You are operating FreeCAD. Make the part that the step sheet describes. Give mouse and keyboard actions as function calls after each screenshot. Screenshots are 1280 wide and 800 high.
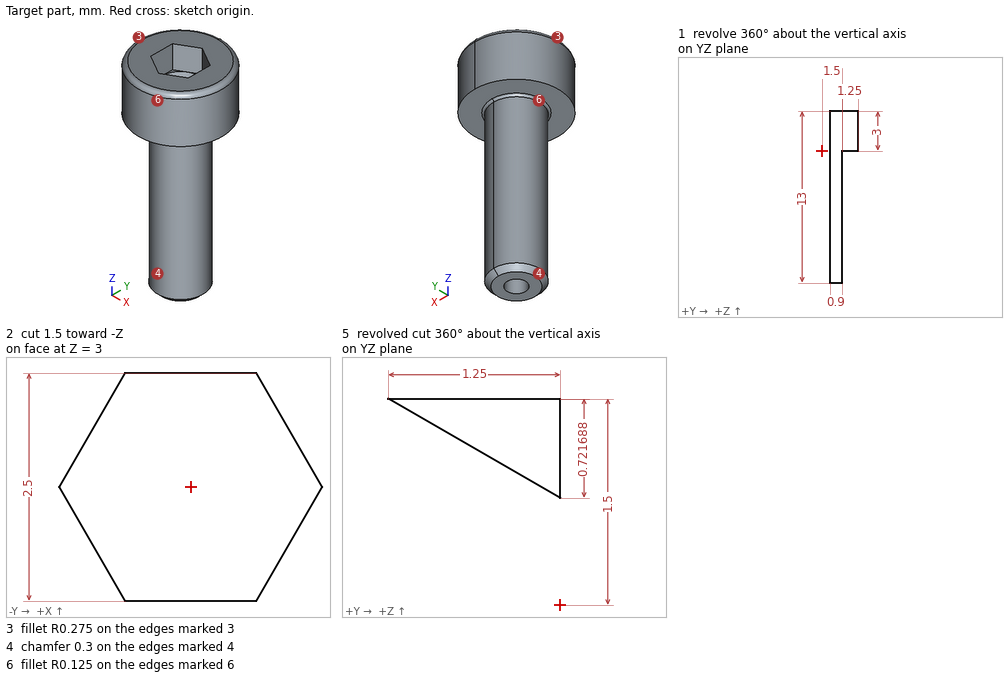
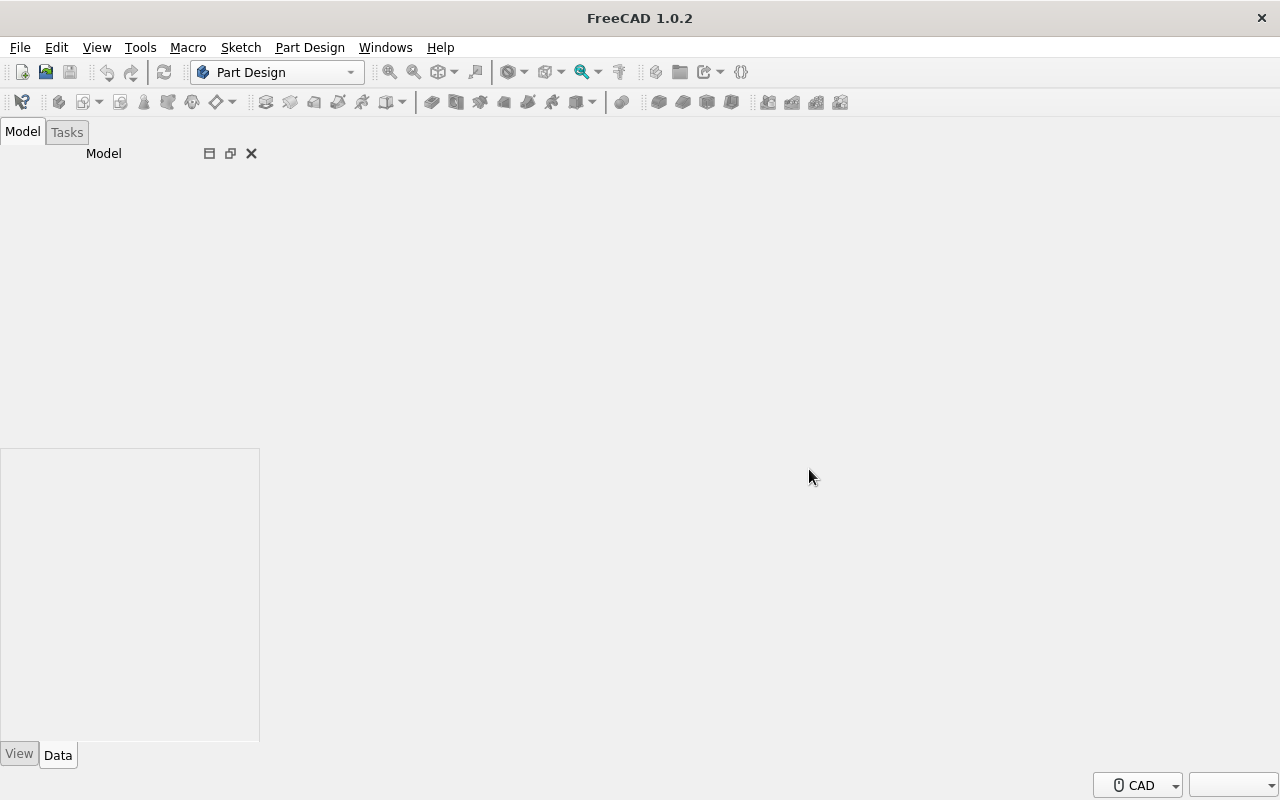
click(22, 72)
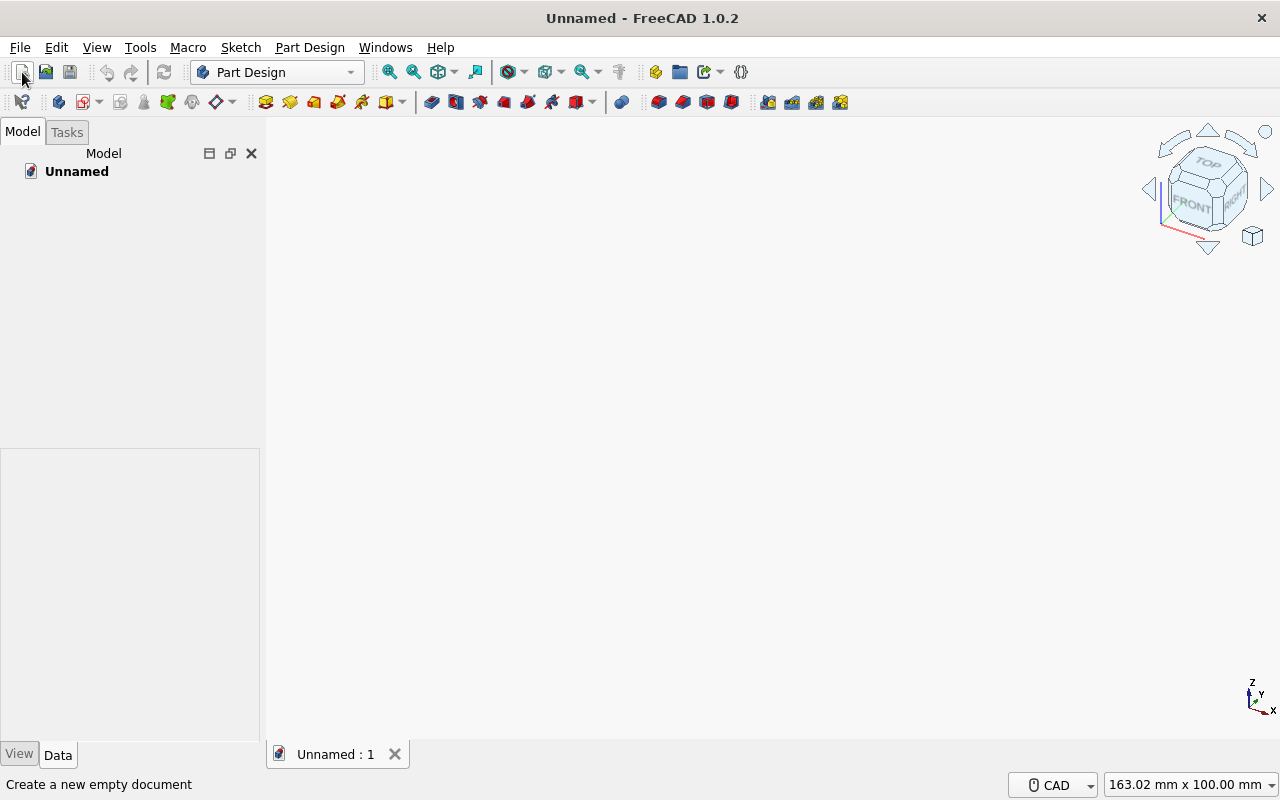
click(84, 102)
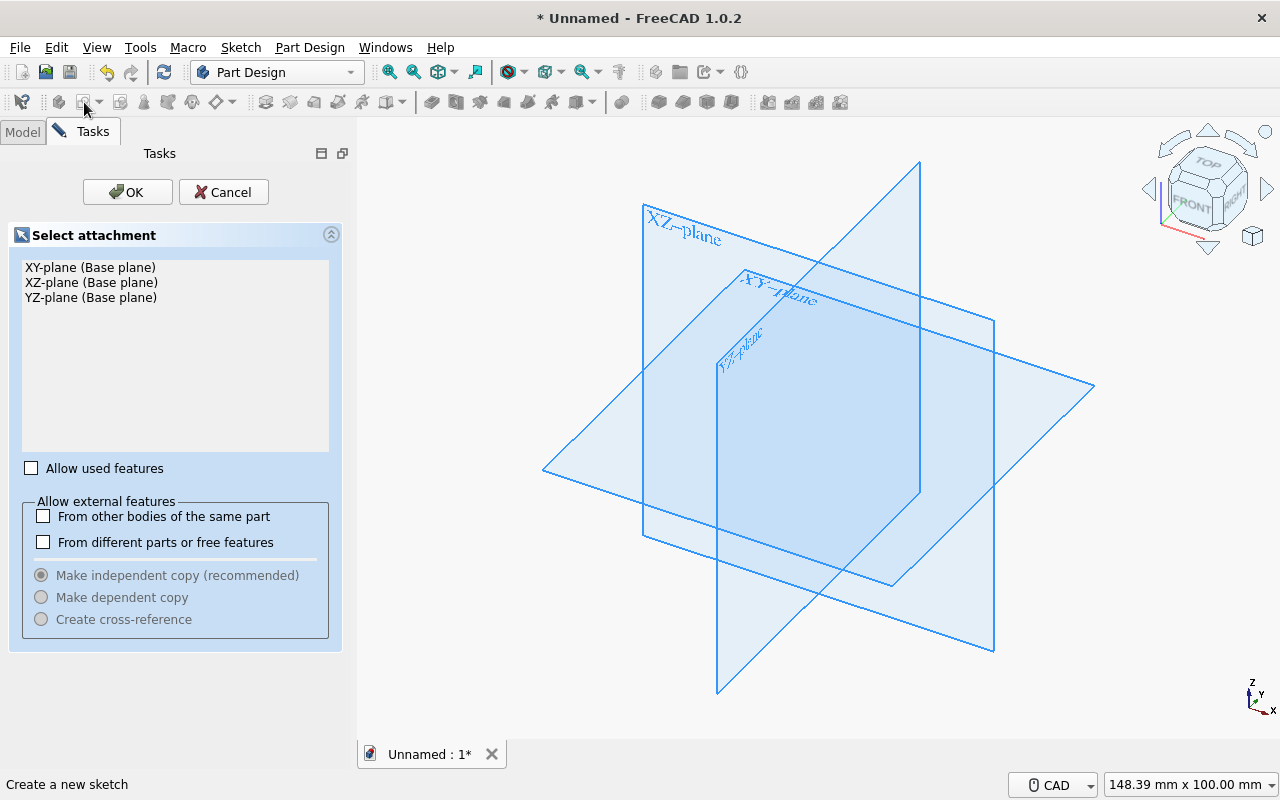
click(82, 298)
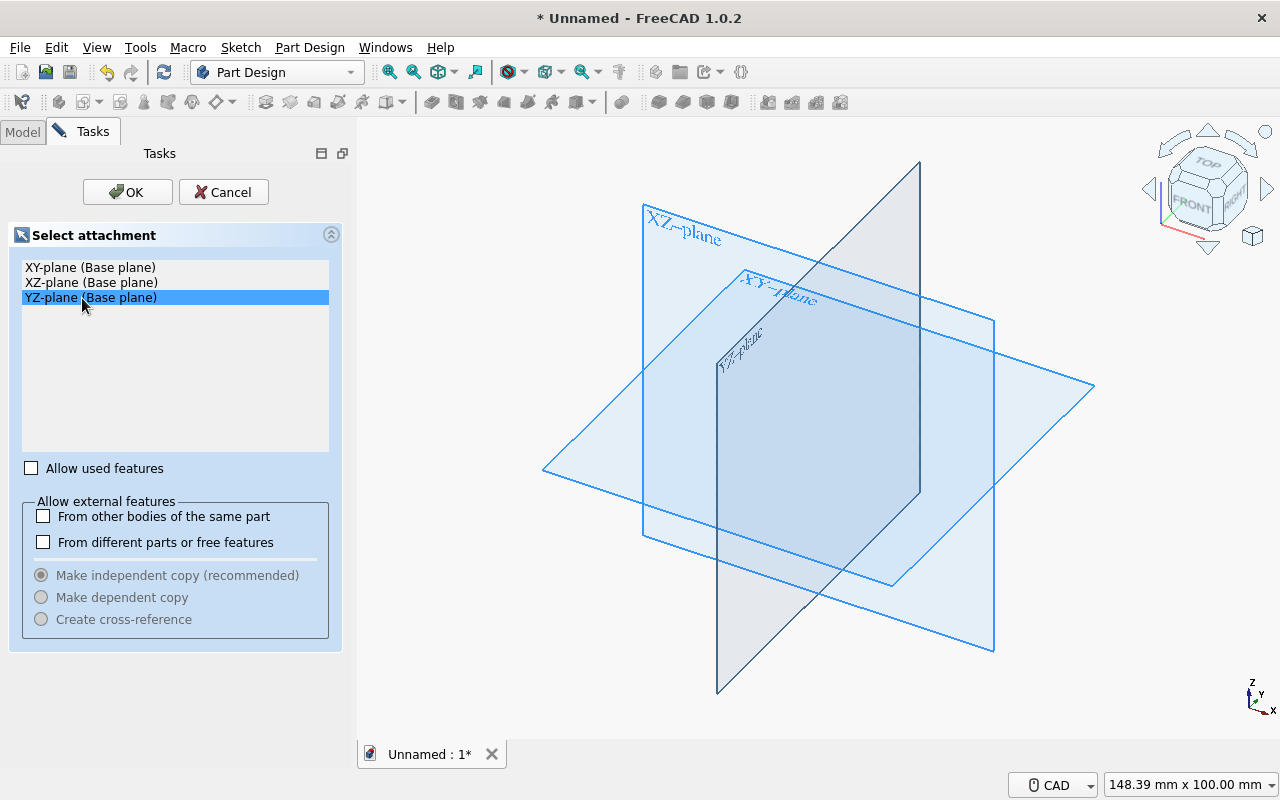
click(128, 192)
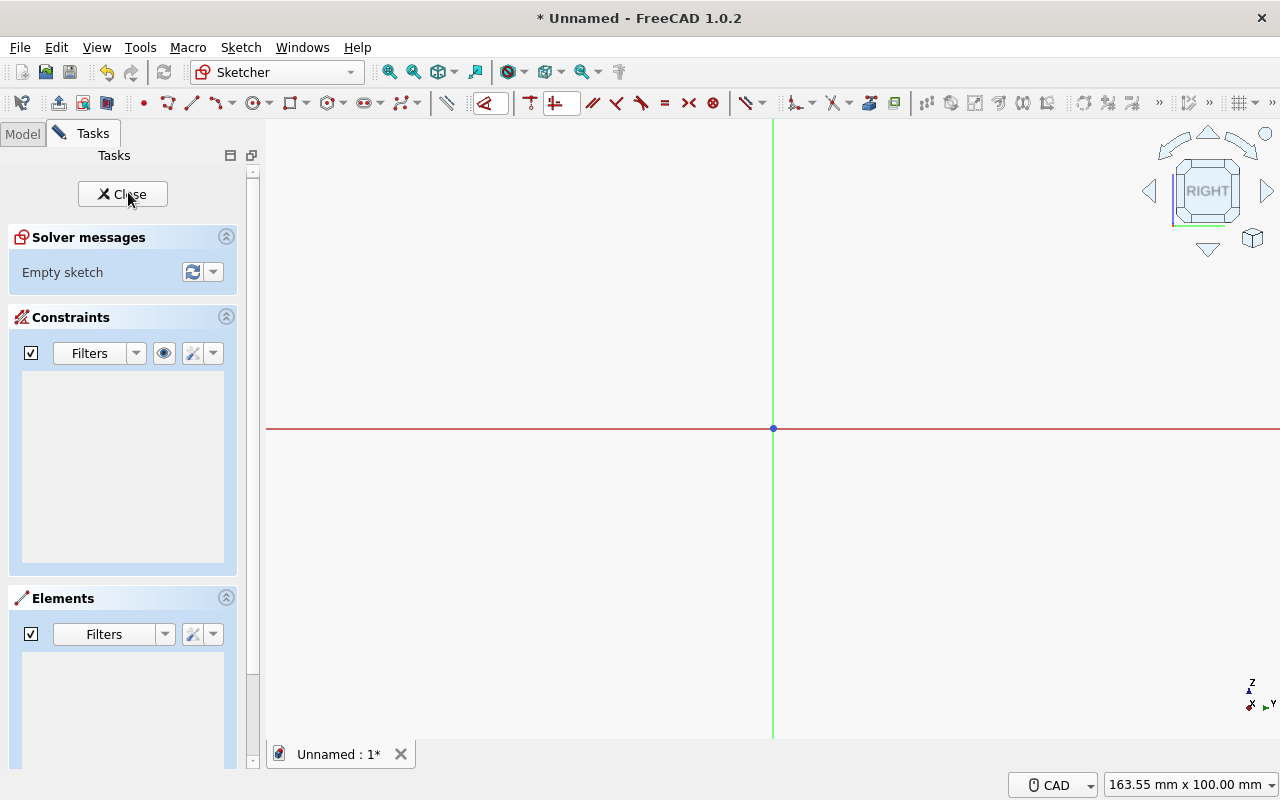
scroll(801, 456, up, 8)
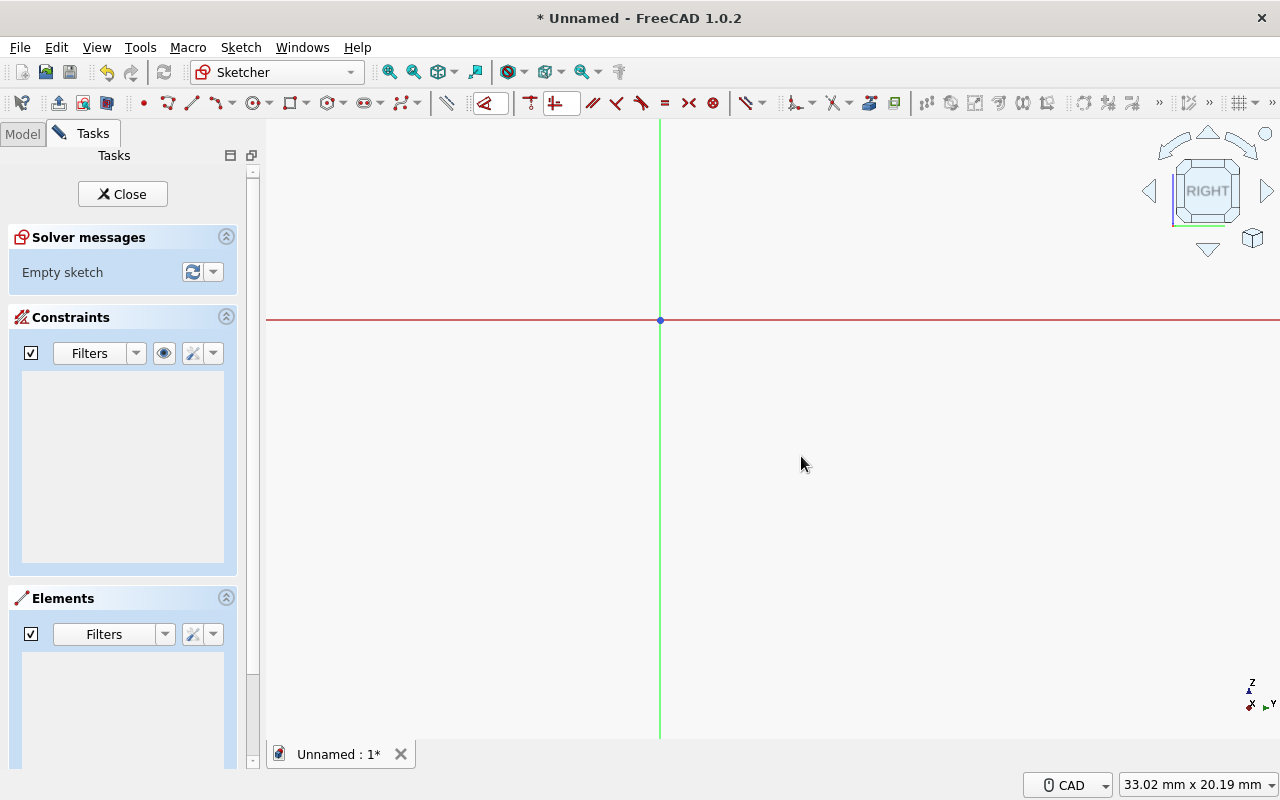
click(168, 104)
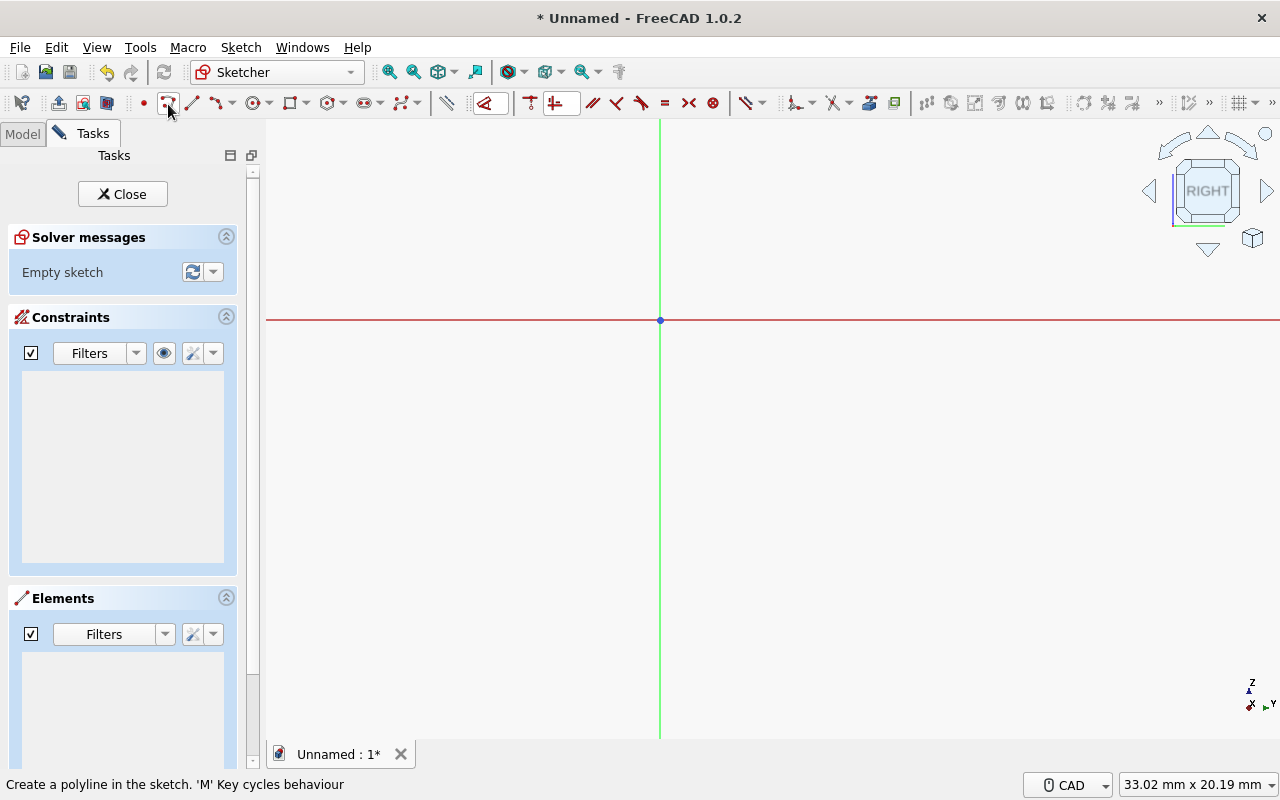
click(706, 320)
click(745, 329)
click(745, 228)
click(679, 228)
click(679, 627)
click(706, 627)
click(706, 320)
key(Escape)
key(Escape)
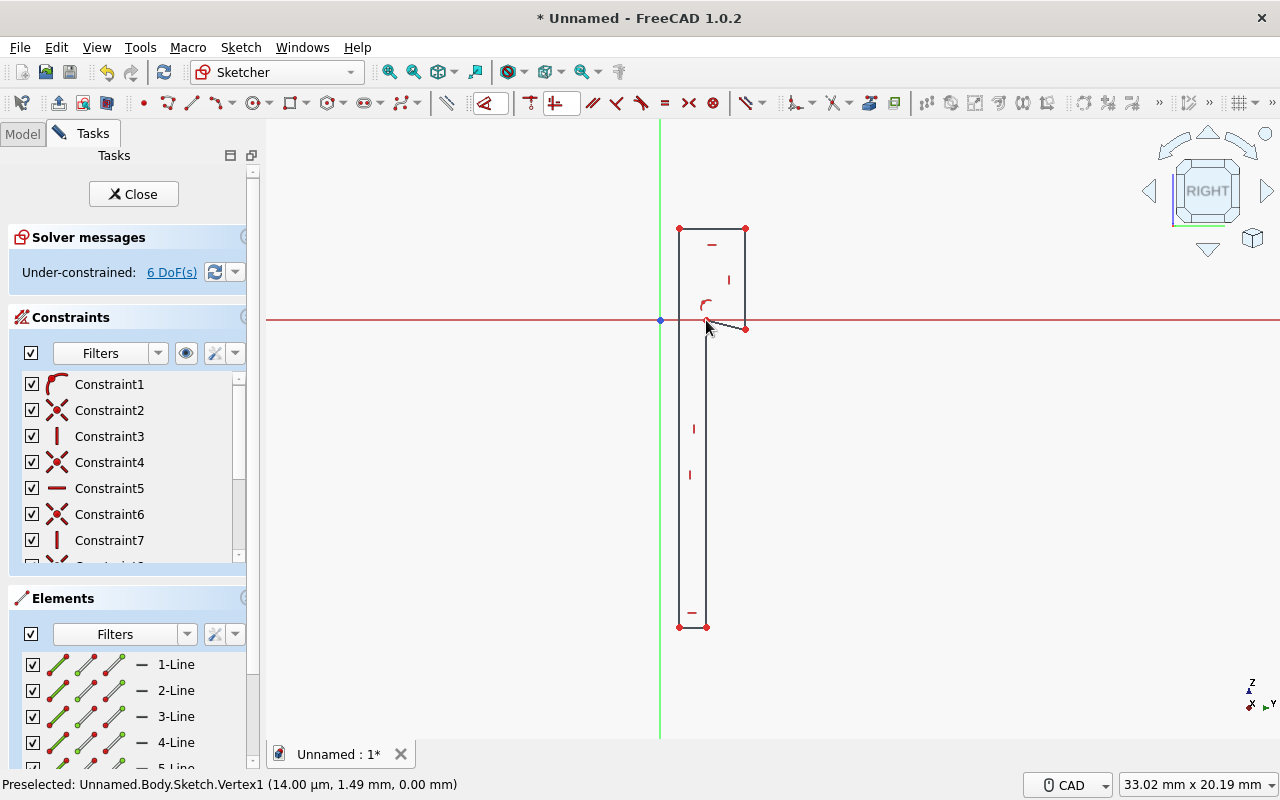
click(718, 323)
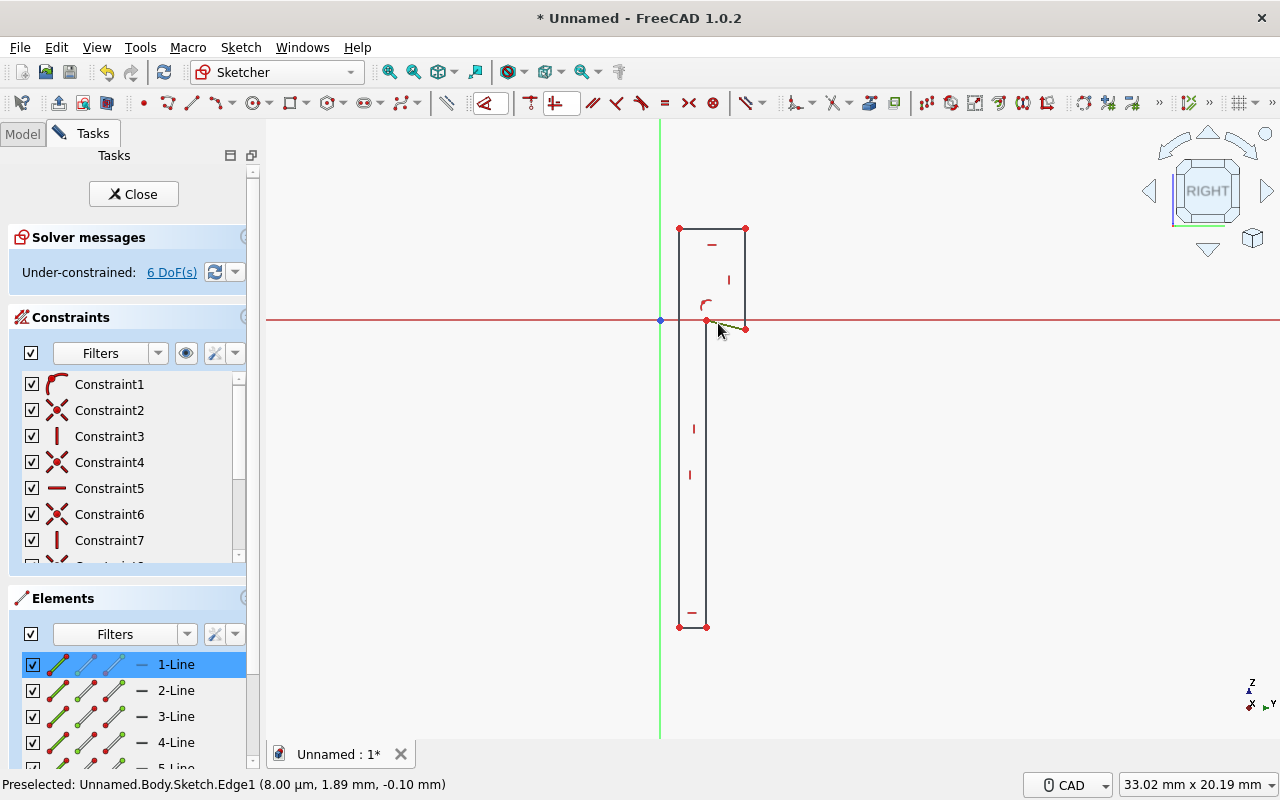
key(h)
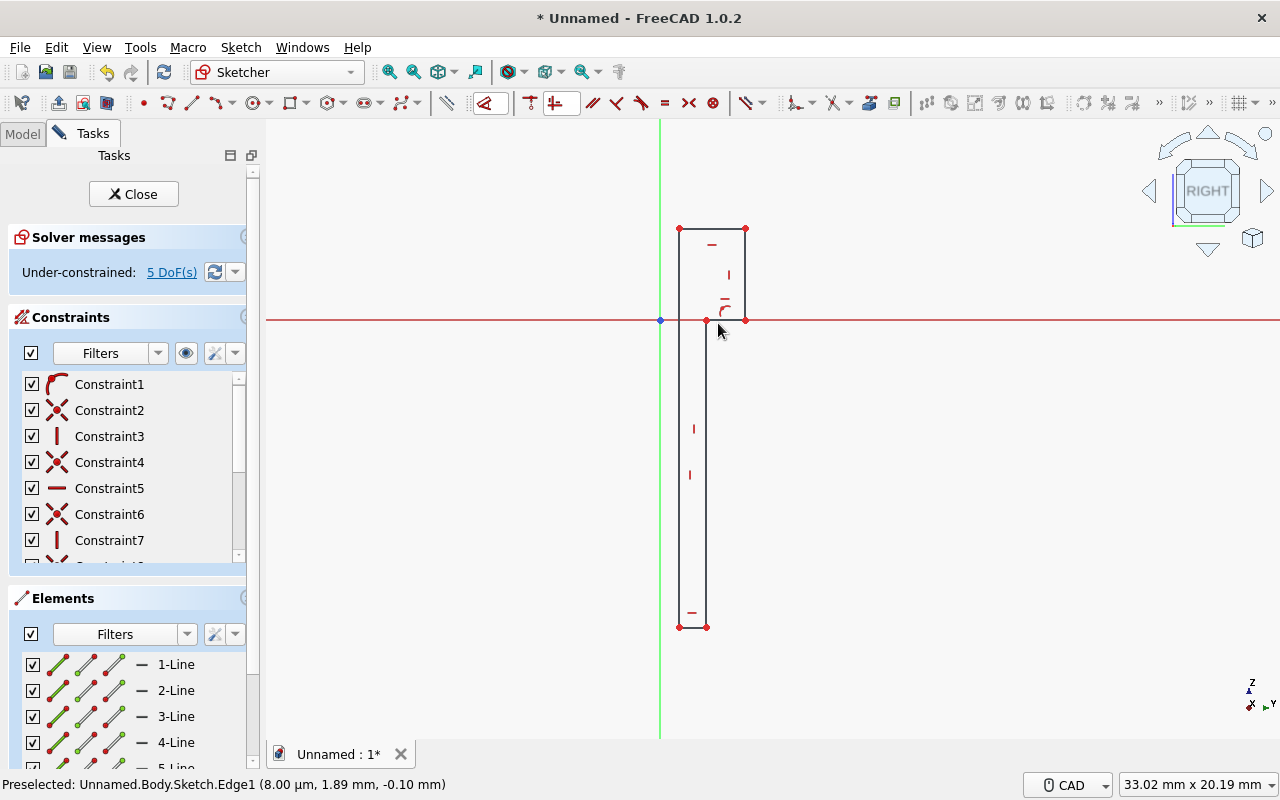
click(745, 293)